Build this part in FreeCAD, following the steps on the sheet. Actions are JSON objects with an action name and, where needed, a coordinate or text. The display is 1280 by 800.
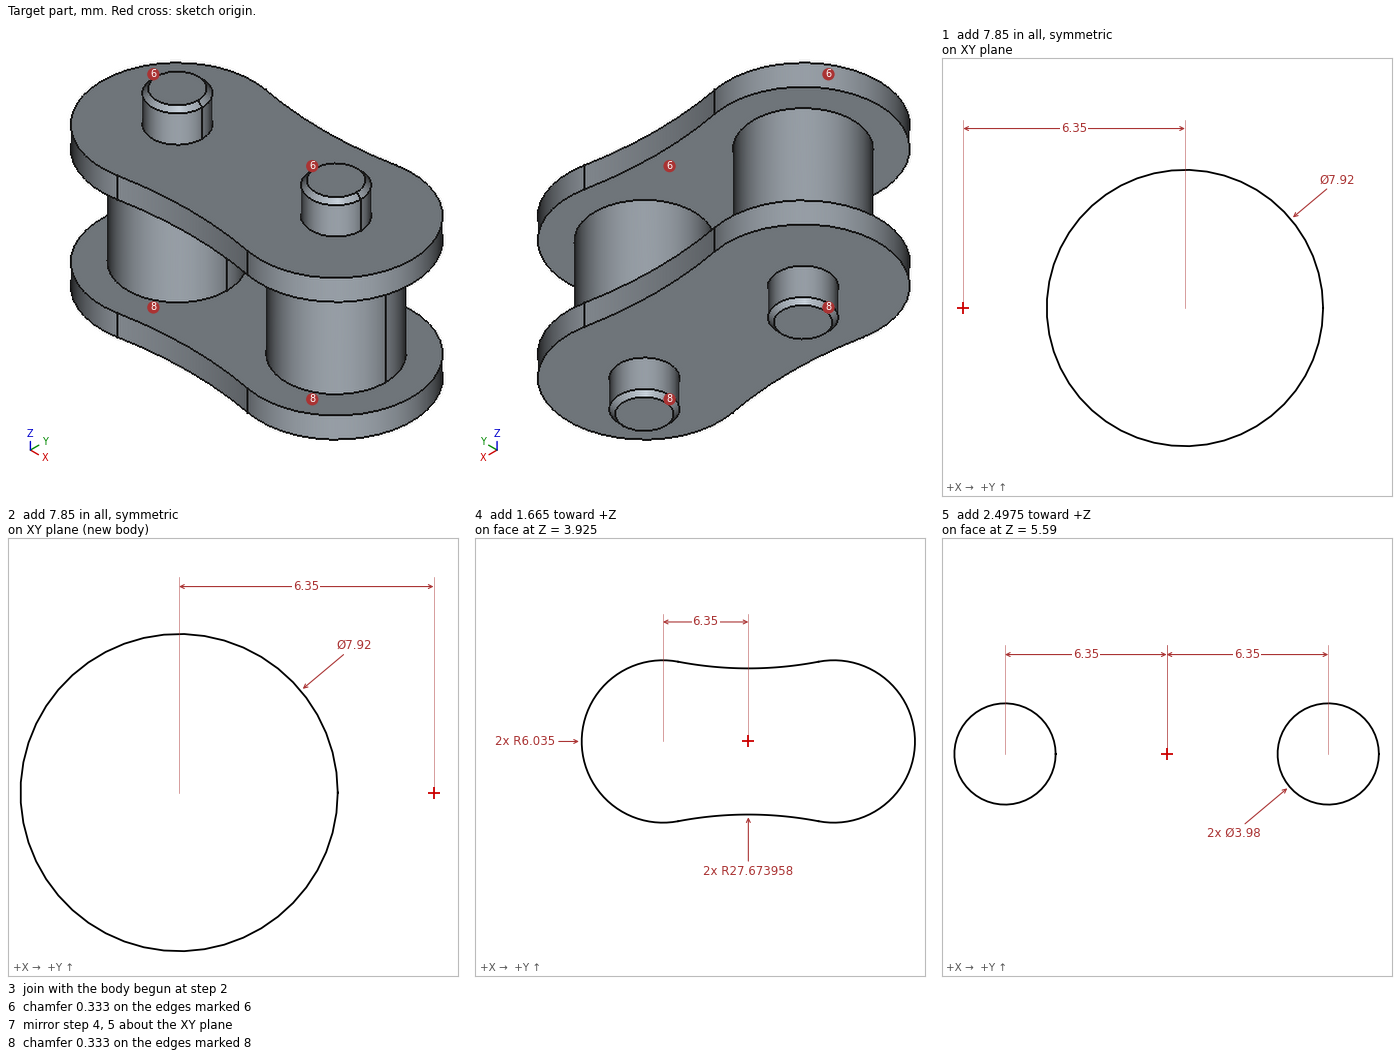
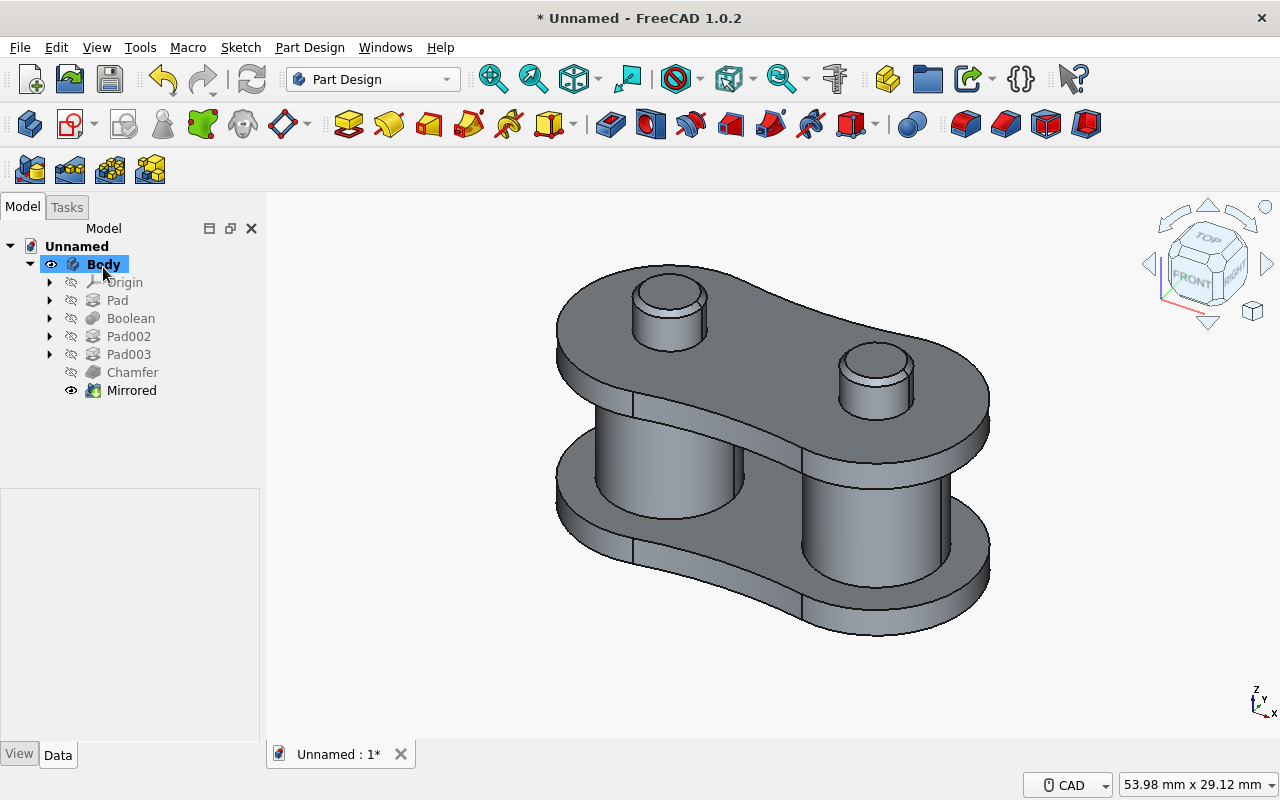
{"action": "key", "text": "0"}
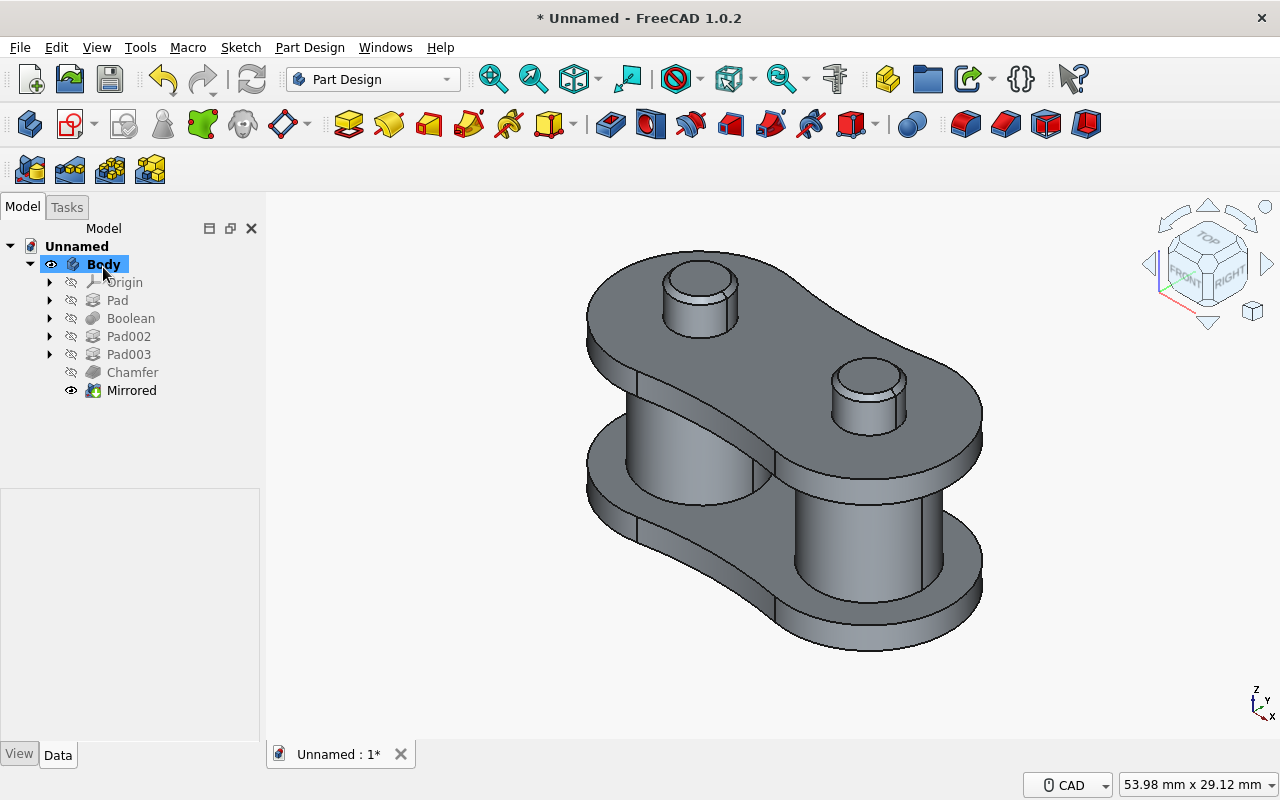
{"action": "left_click", "coordinate": [494, 80]}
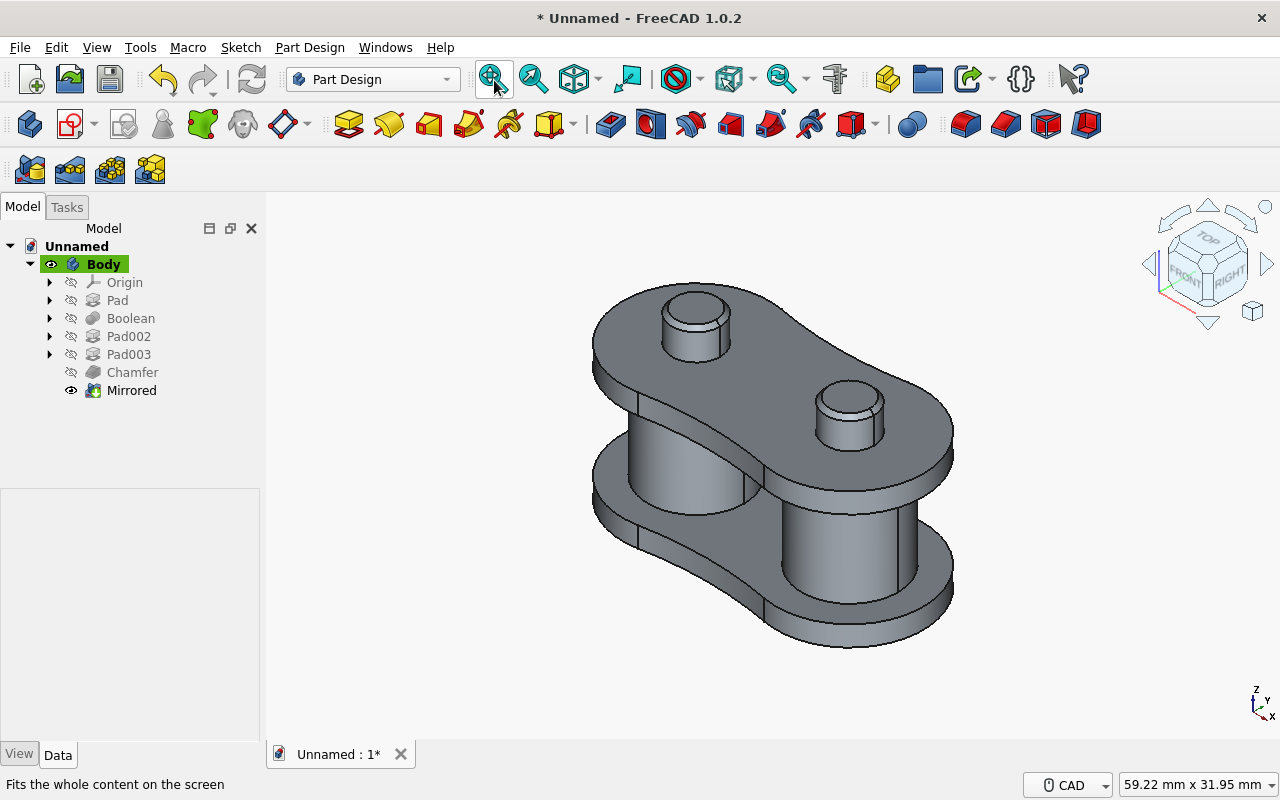
{"action": "key", "text": "2"}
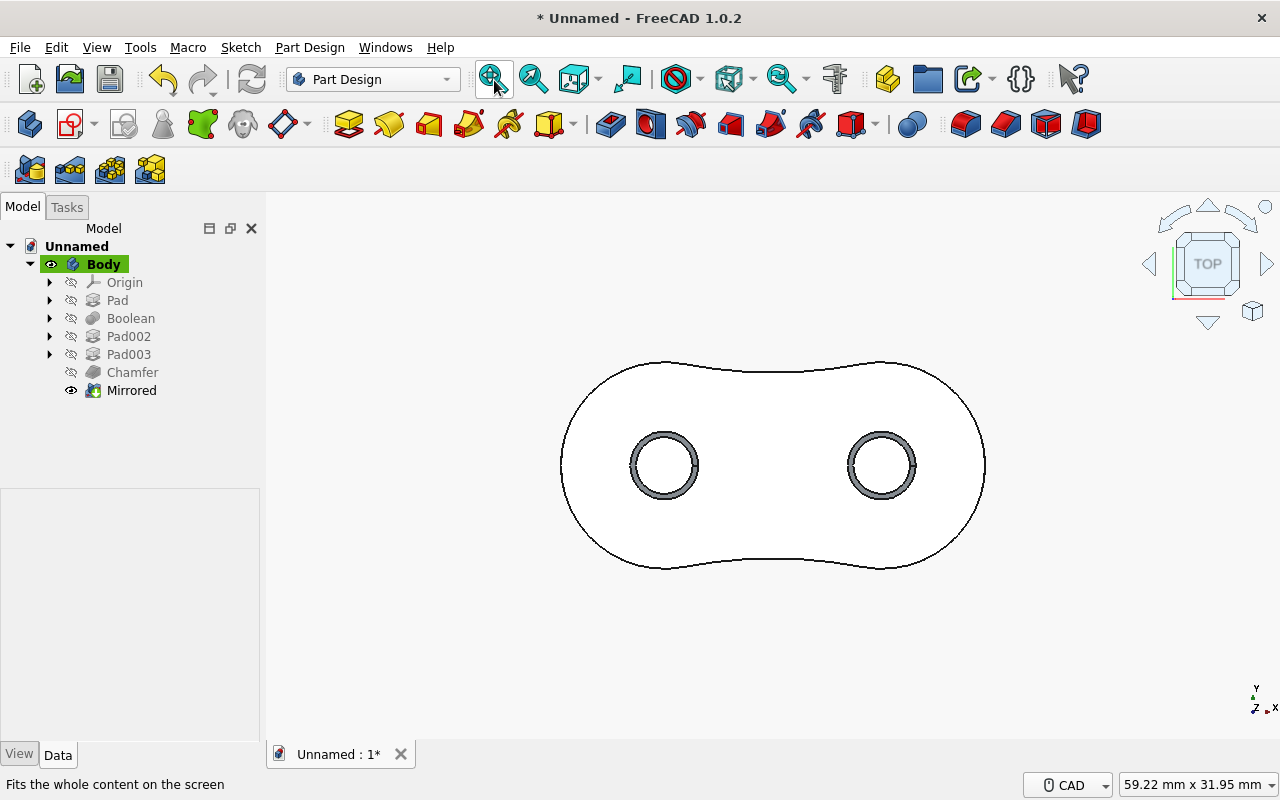
{"action": "left_click", "coordinate": [494, 80]}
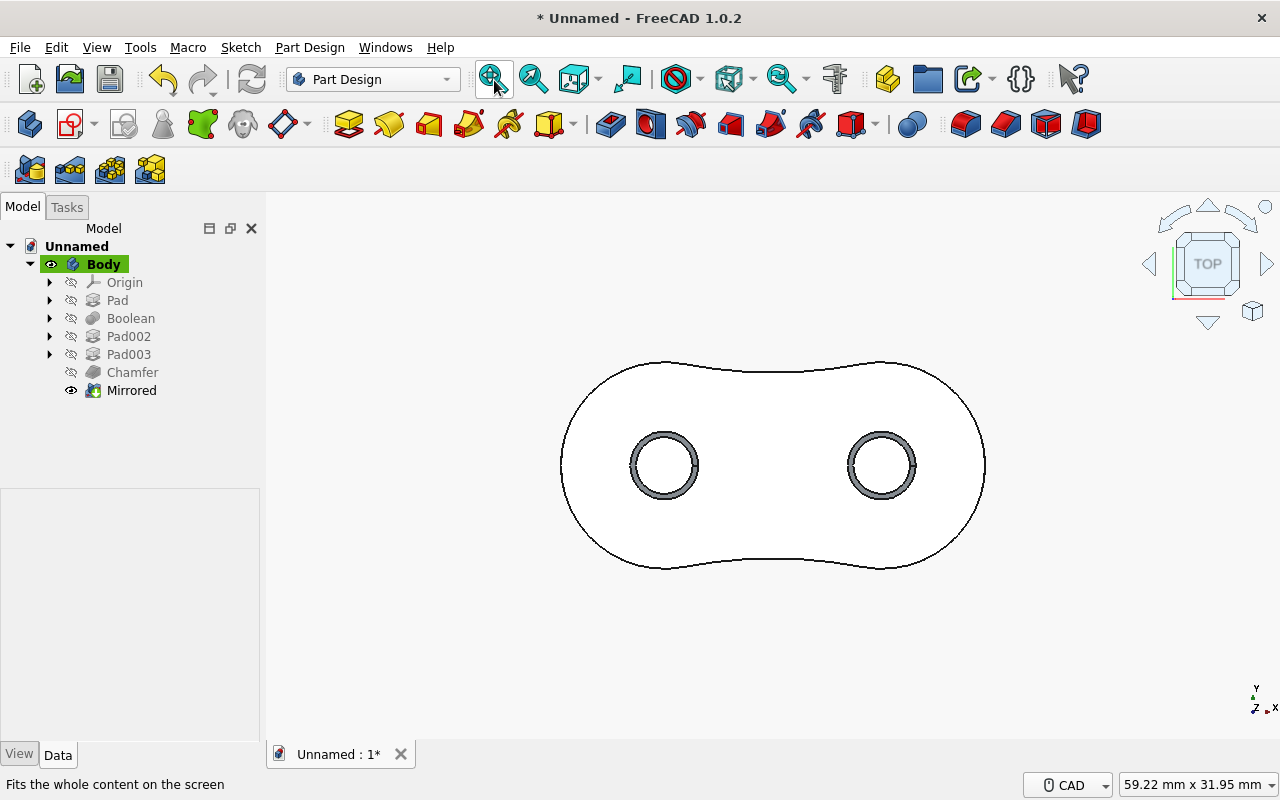
{"action": "key", "text": "1"}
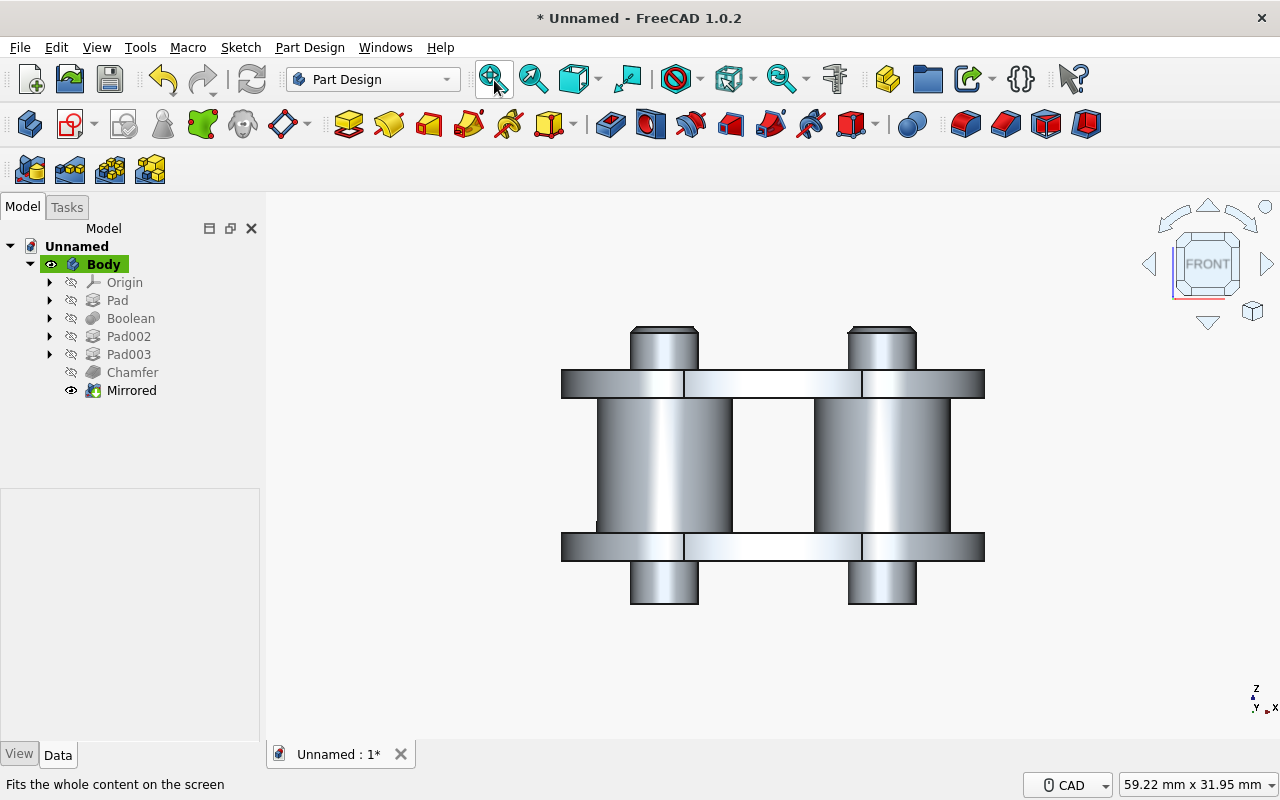
{"action": "left_click", "coordinate": [848, 603]}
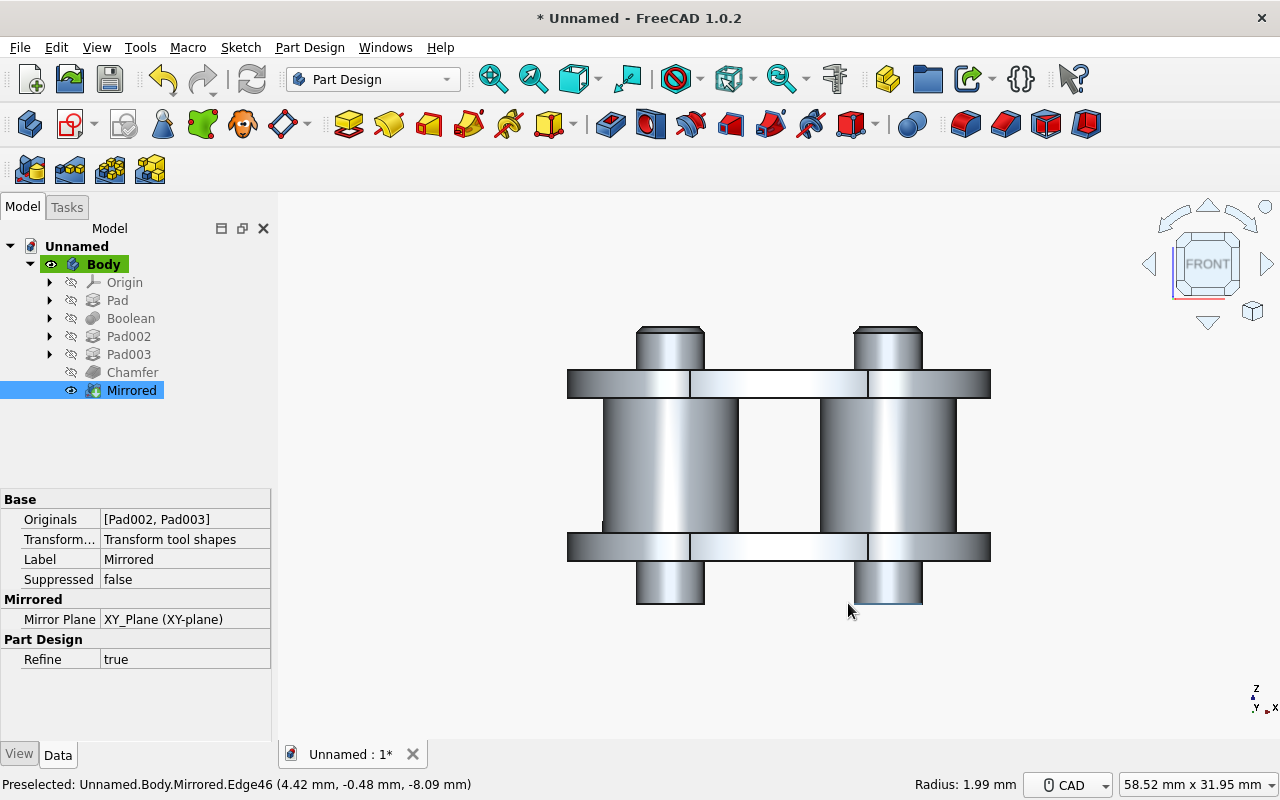
{"action": "left_click", "coordinate": [643, 603], "text": "ctrl"}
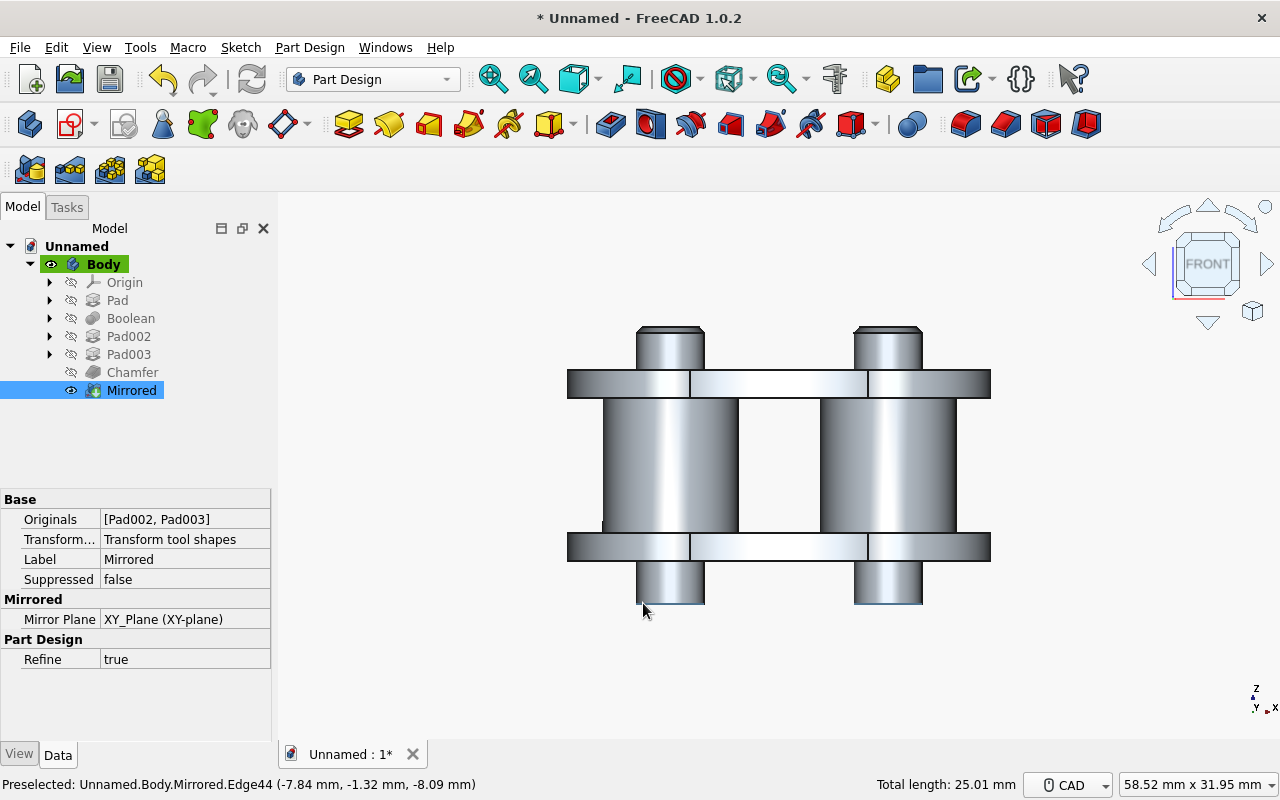
{"action": "left_click", "coordinate": [1006, 124]}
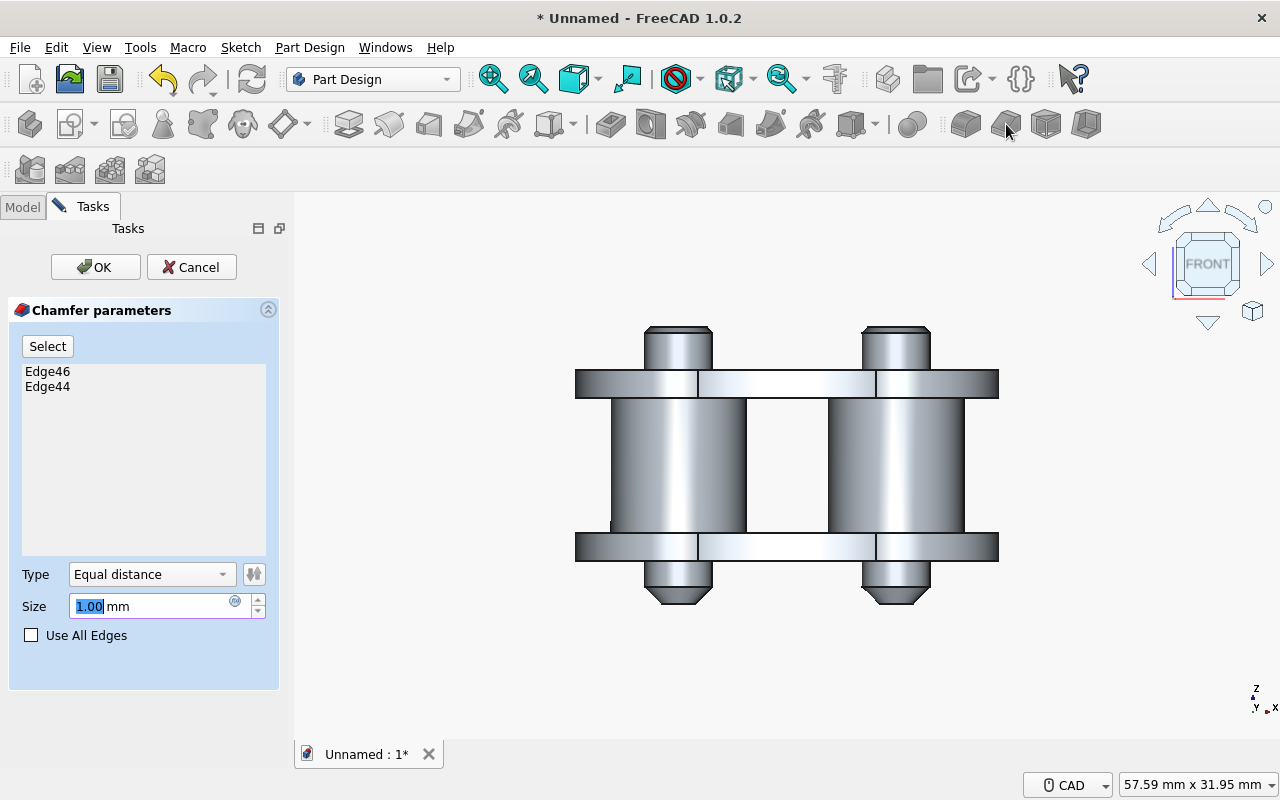
{"action": "type", "text": "0.333"}
{"action": "key", "text": "Tab"}